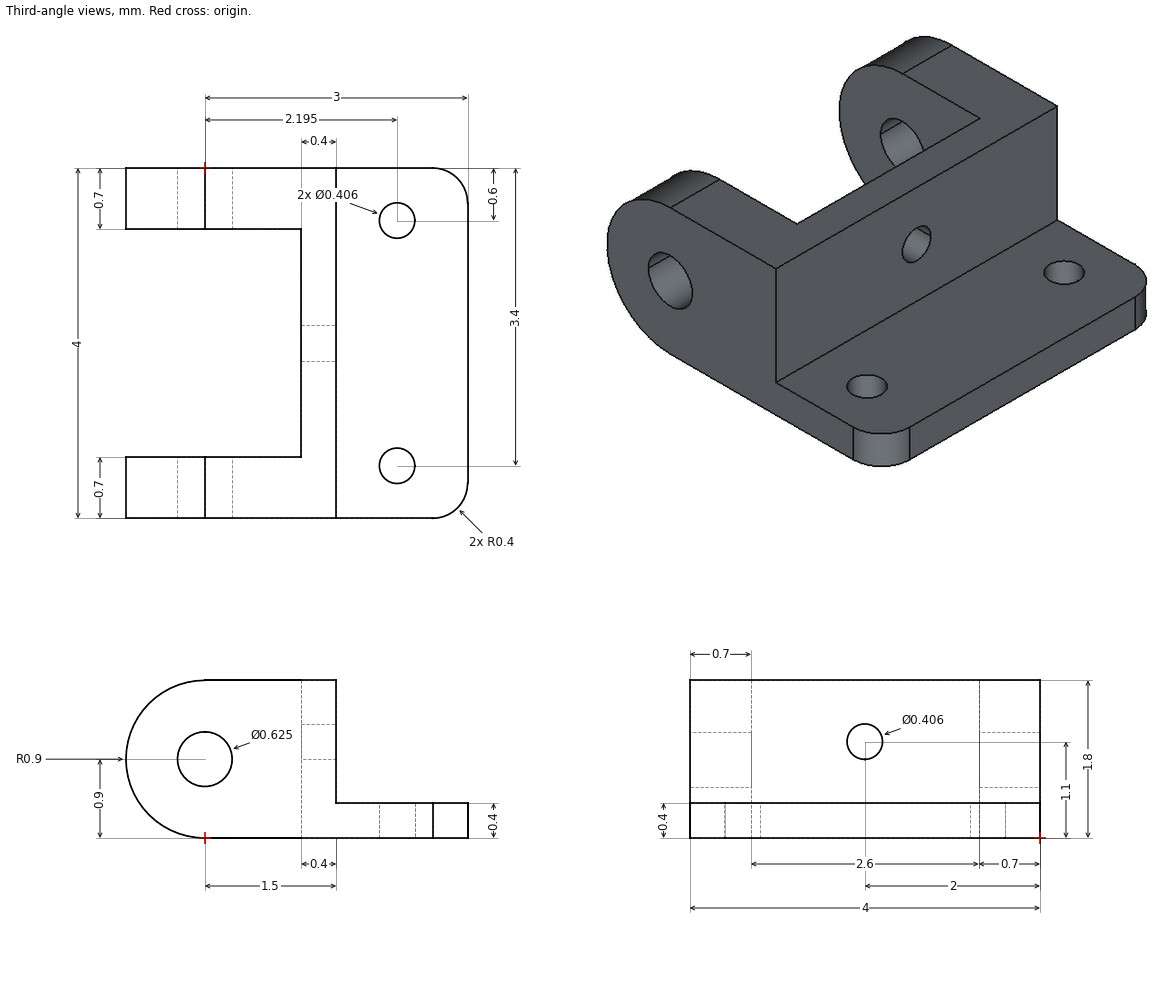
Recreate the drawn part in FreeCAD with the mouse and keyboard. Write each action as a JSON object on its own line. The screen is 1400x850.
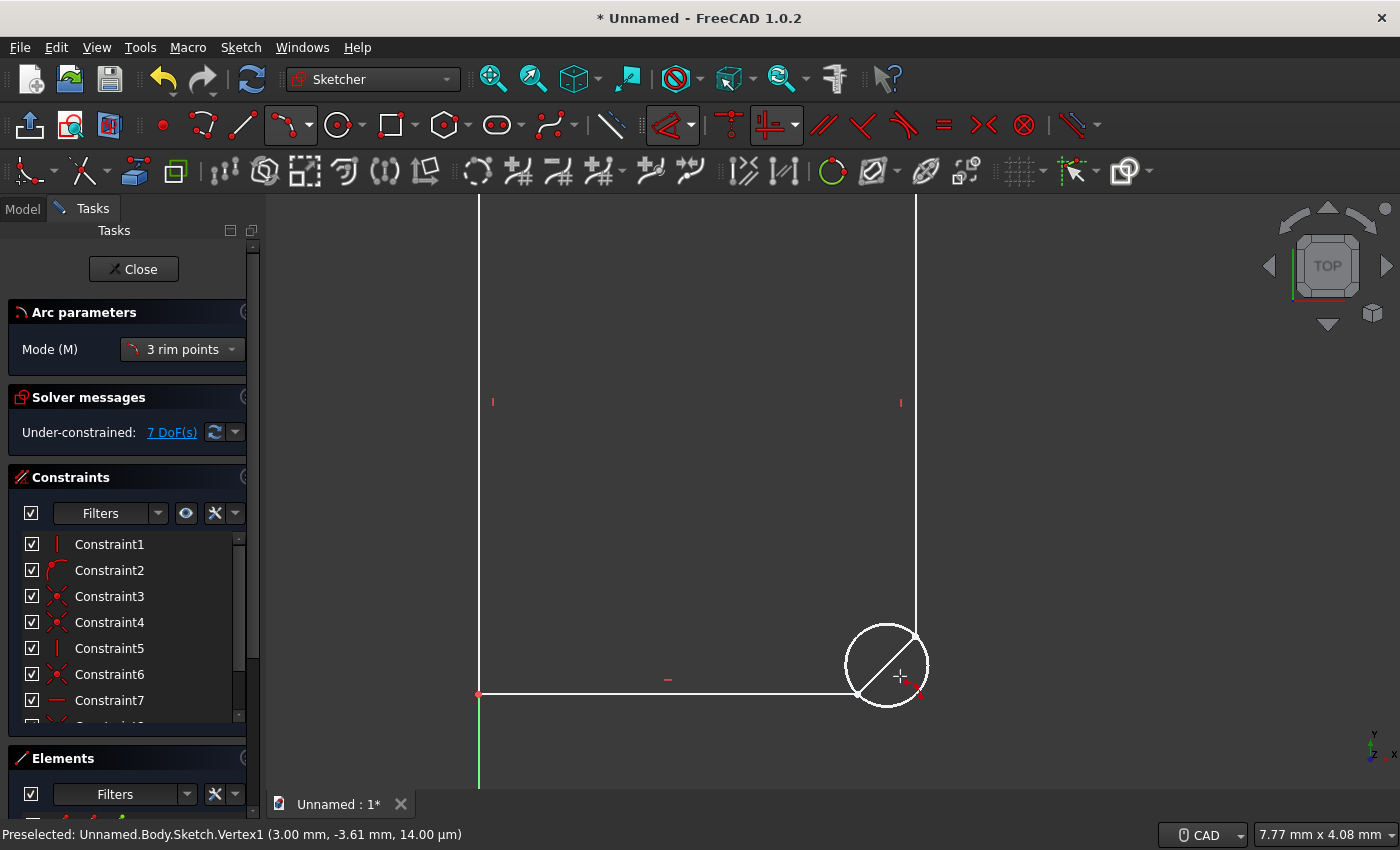
{"action": "left_click", "coordinate": [899, 675]}
{"action": "key", "text": "Escape"}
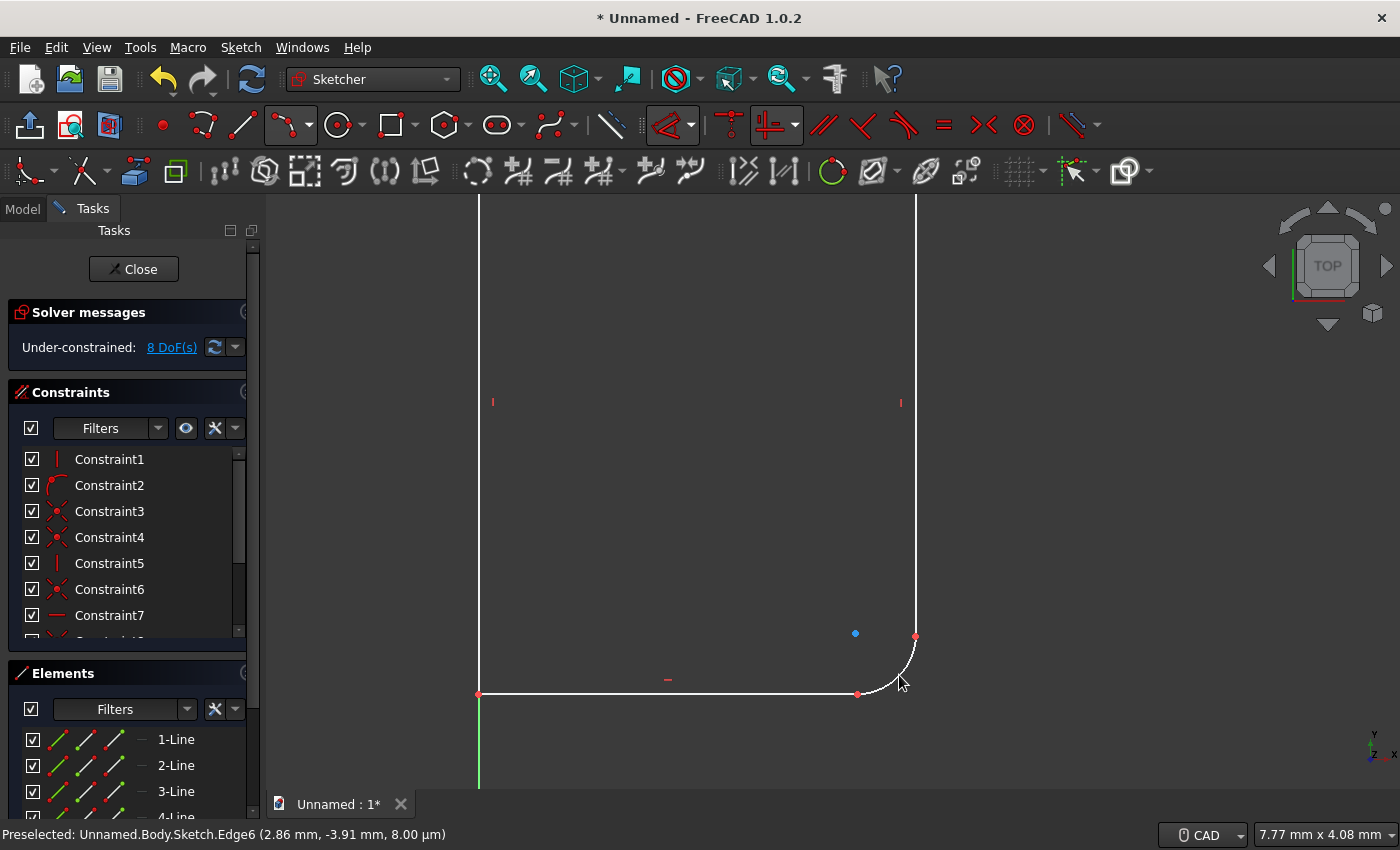
{"action": "left_click", "coordinate": [916, 496]}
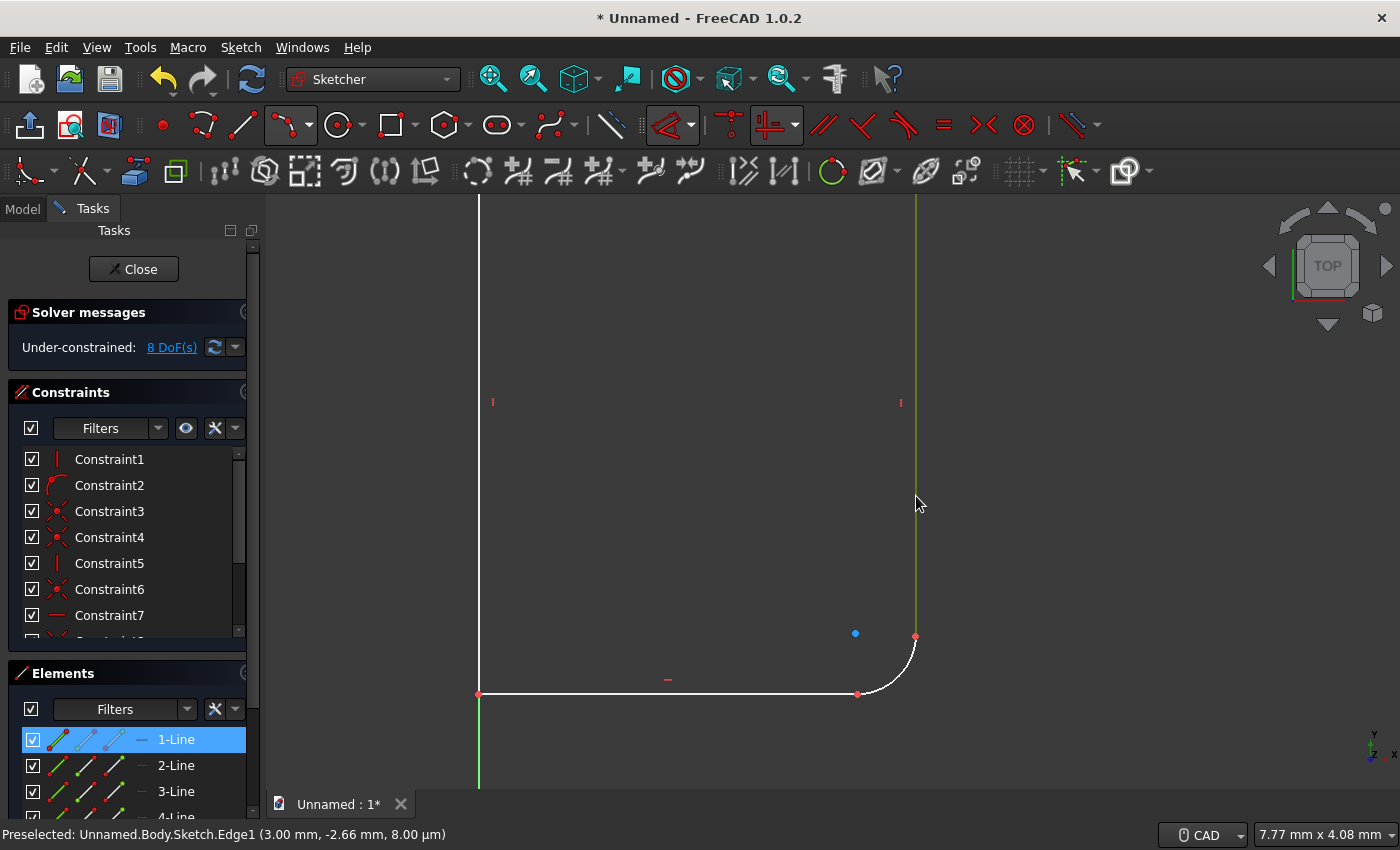
{"action": "scroll", "coordinate": [900, 676], "scroll_direction": "down", "scroll_amount": 2}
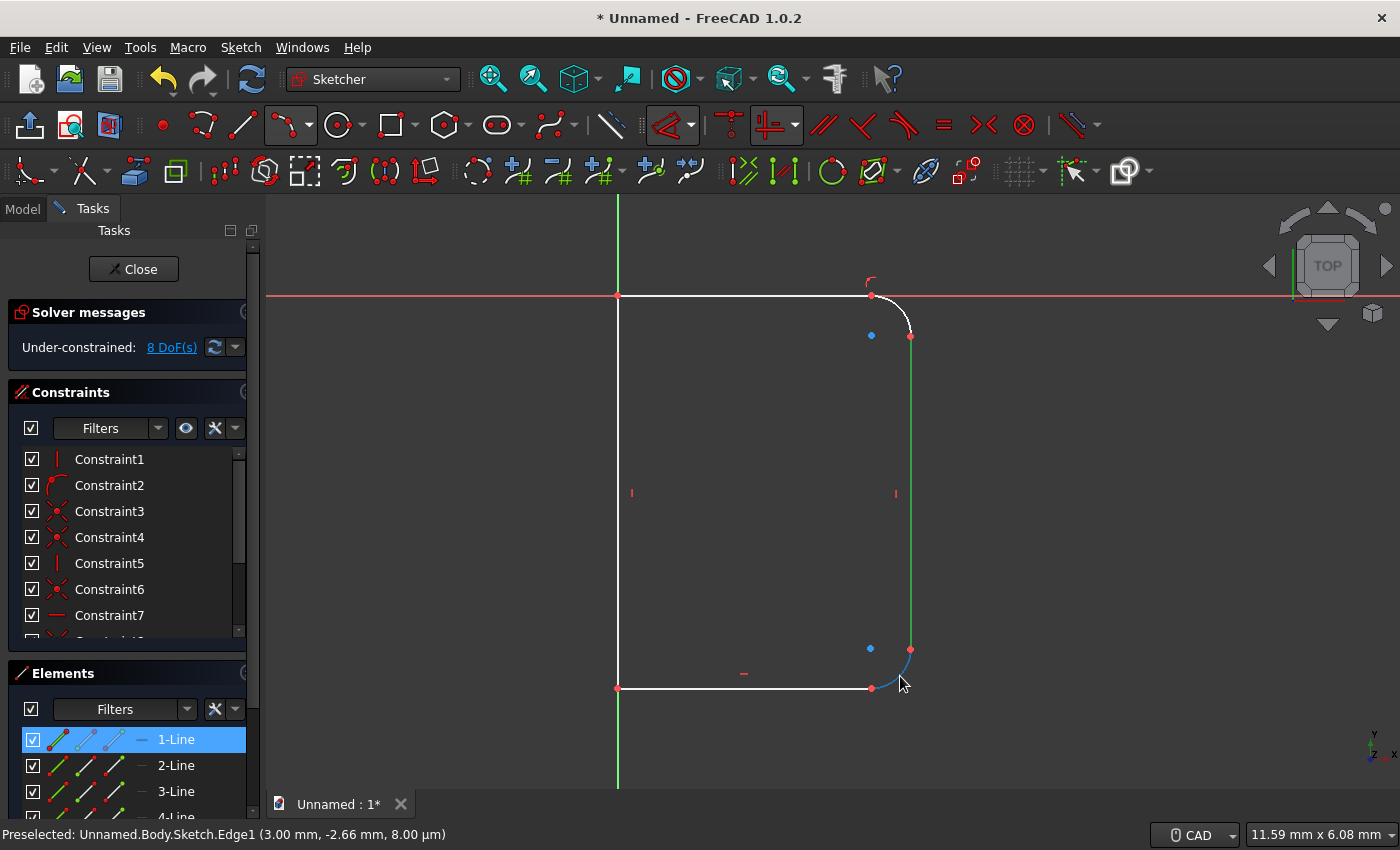
{"action": "left_click", "coordinate": [907, 318]}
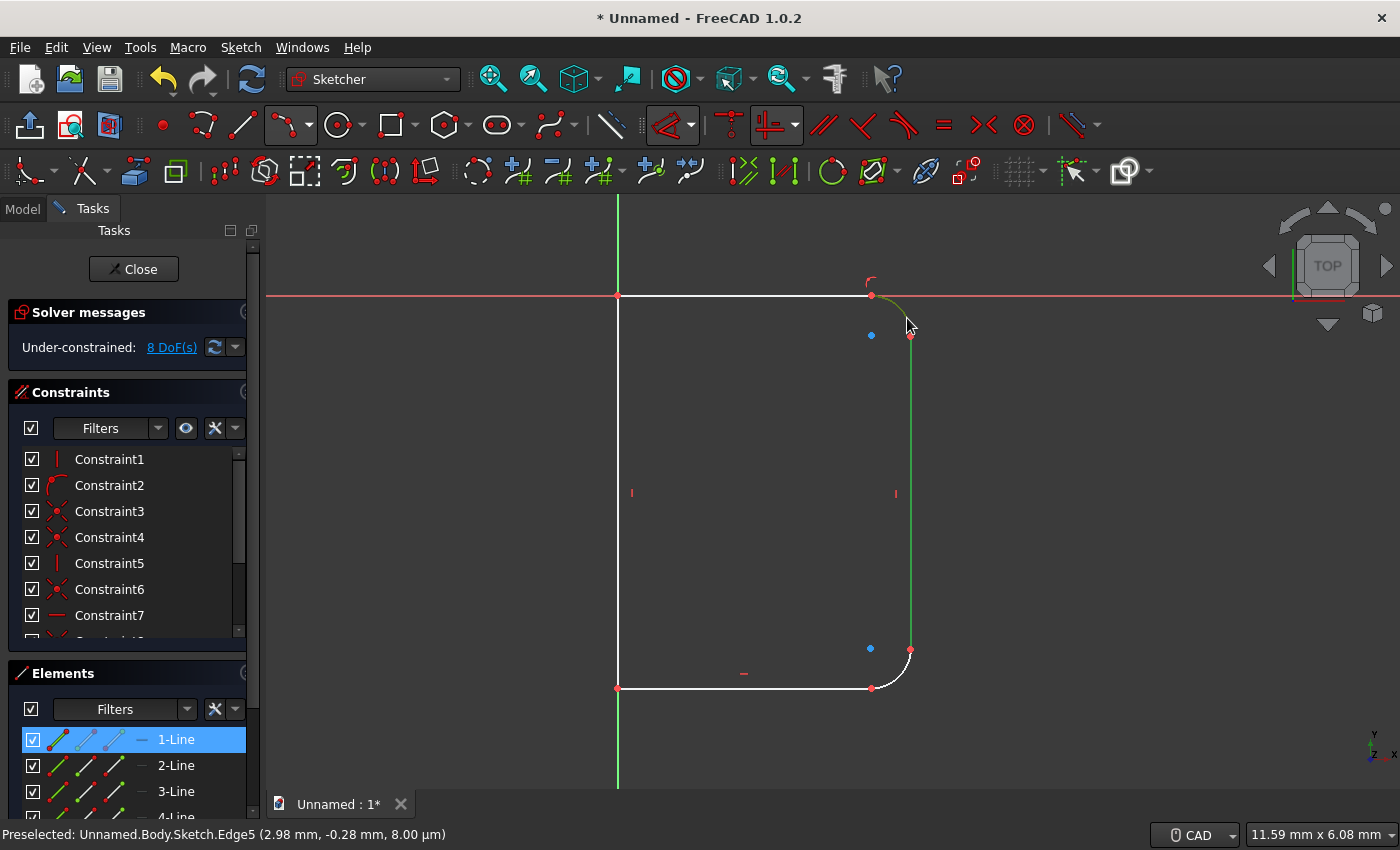
{"action": "left_click", "coordinate": [904, 126]}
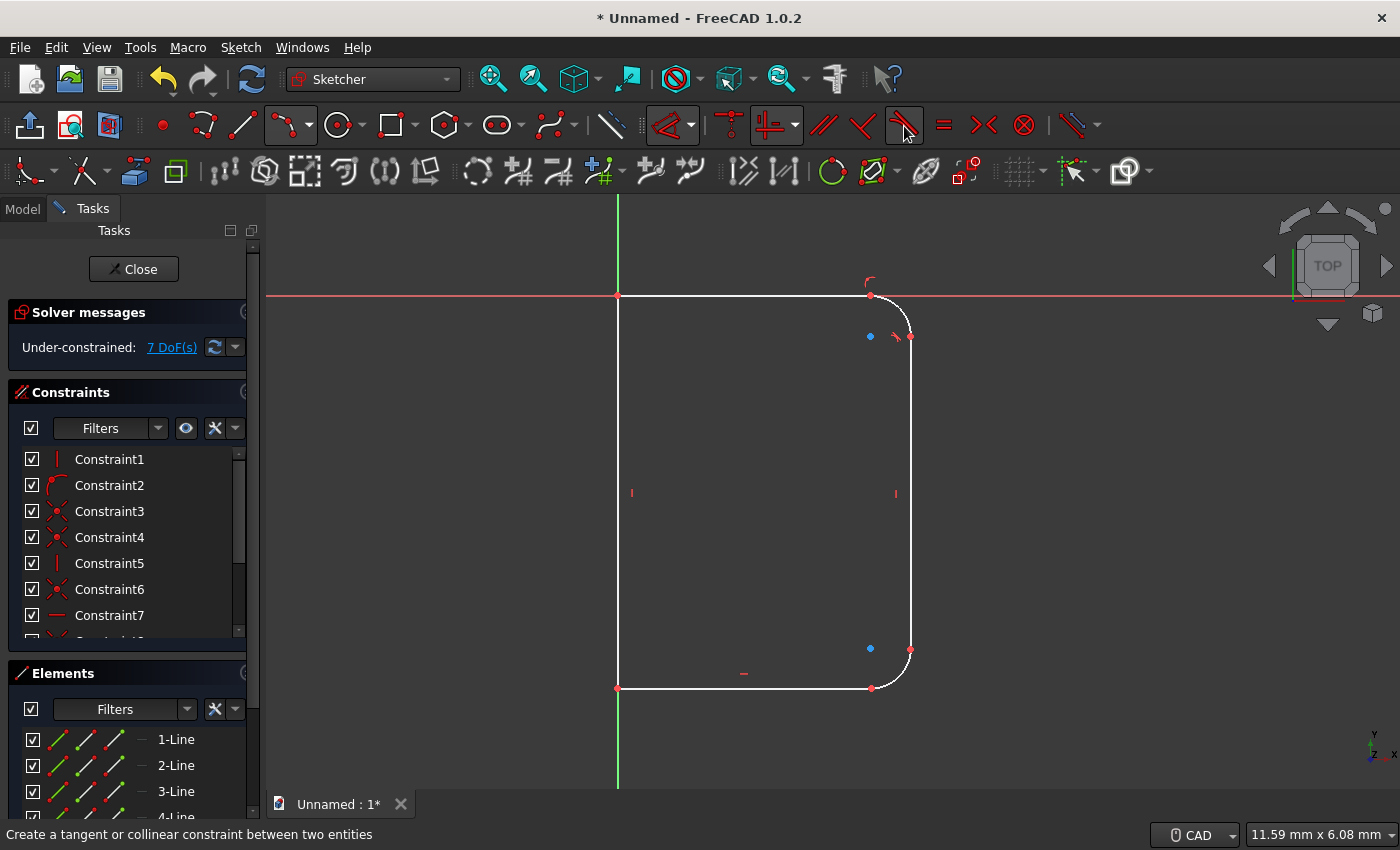
{"action": "left_click", "coordinate": [911, 556]}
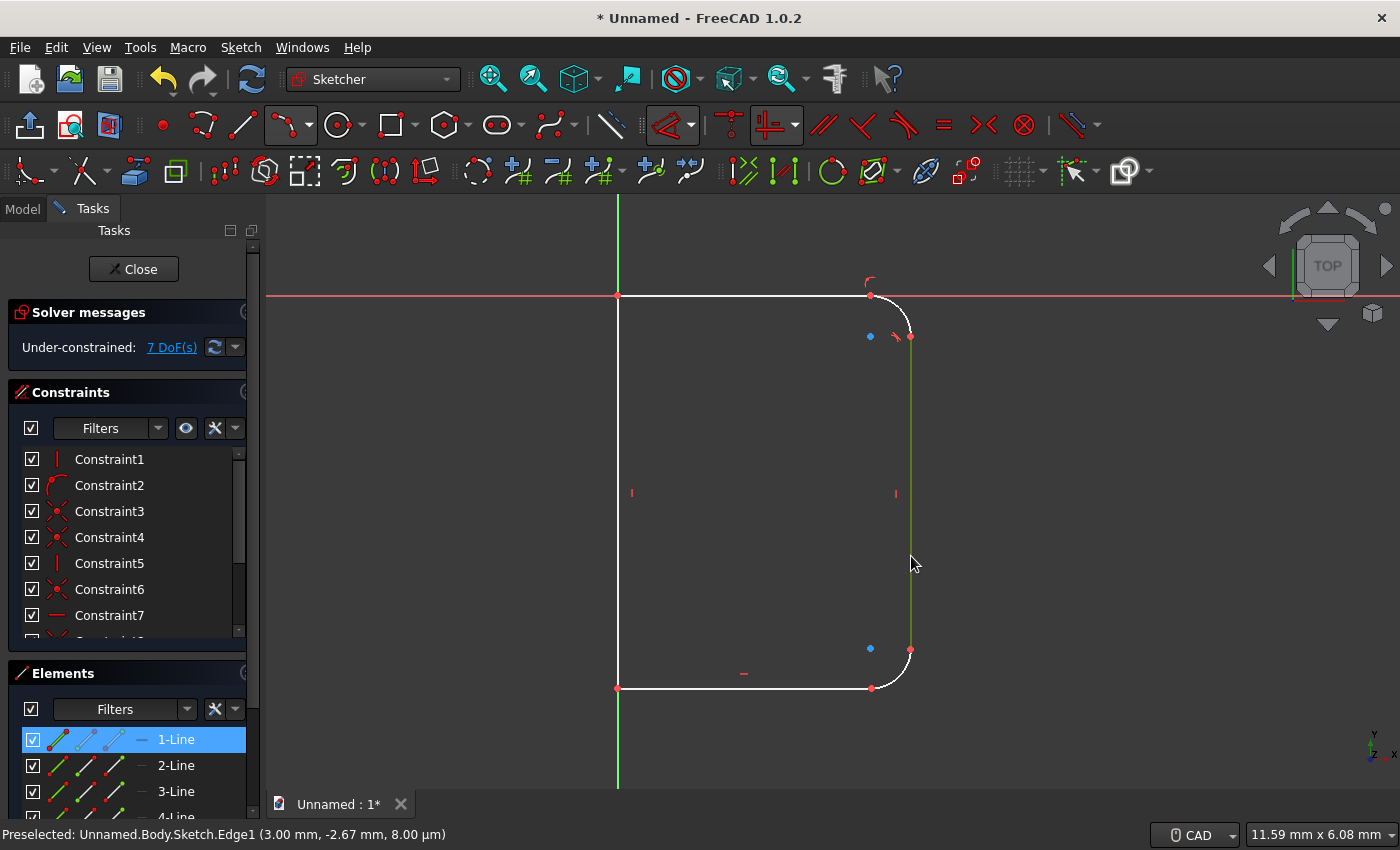
{"action": "left_click", "coordinate": [889, 684]}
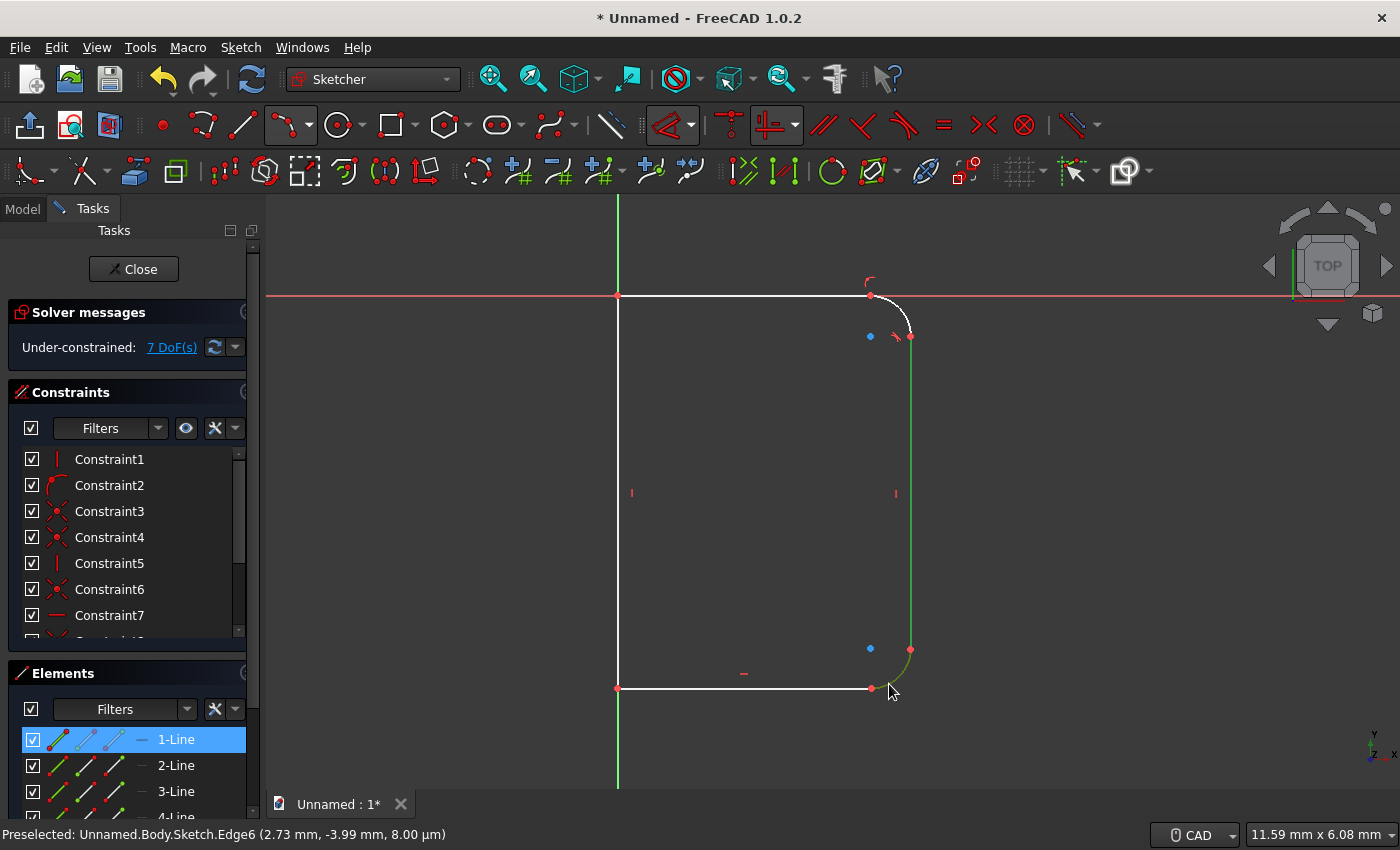
{"action": "key", "text": "t"}